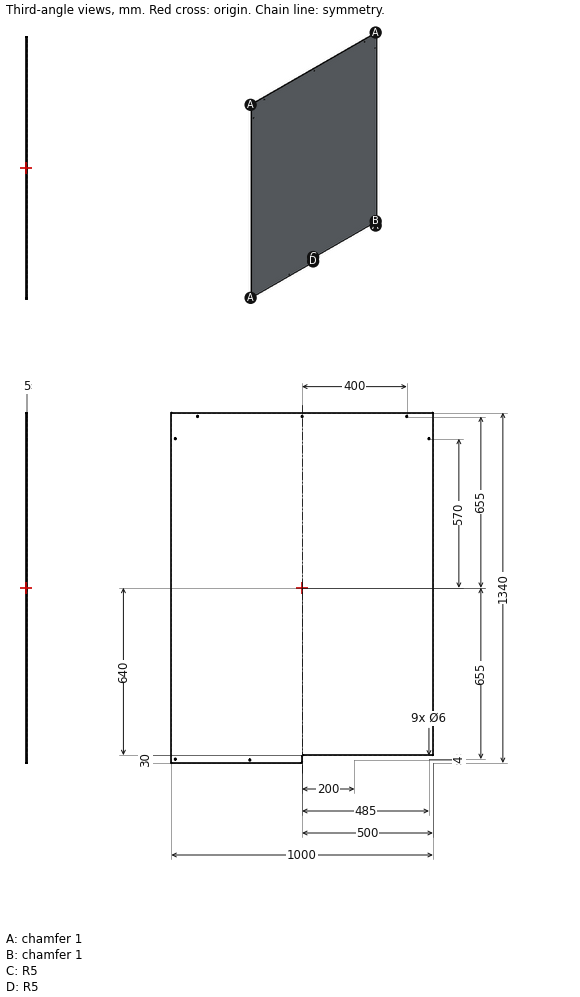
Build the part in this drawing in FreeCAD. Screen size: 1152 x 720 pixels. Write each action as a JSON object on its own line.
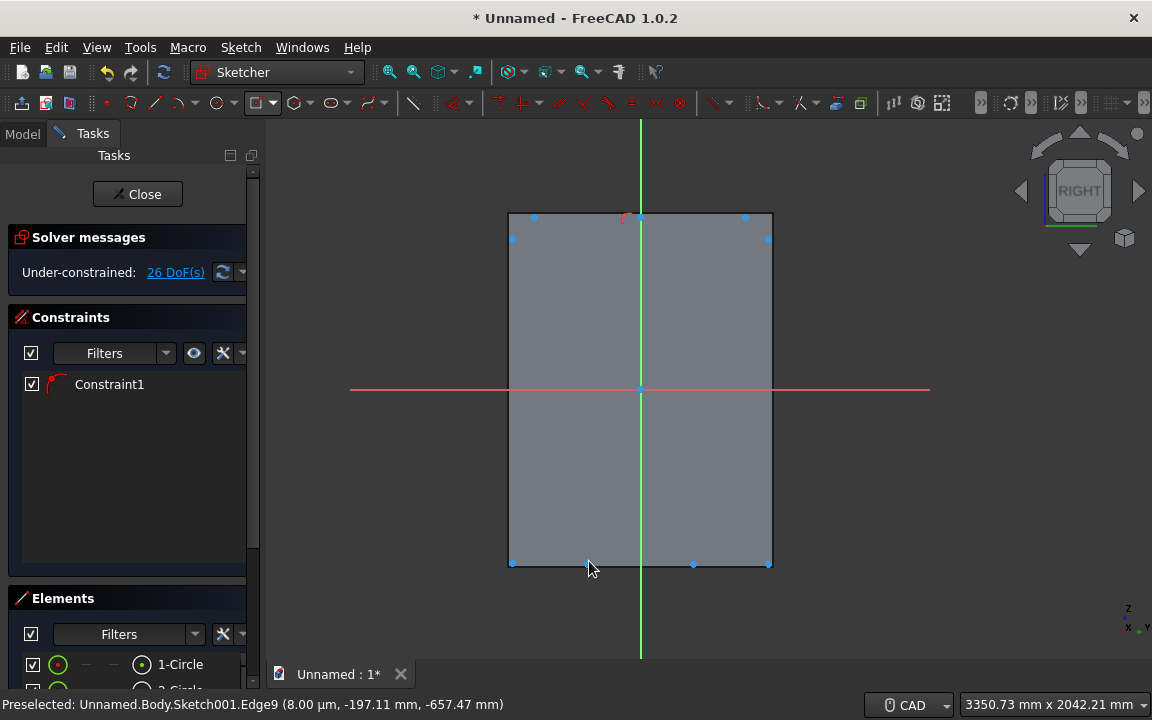
{"action": "scroll", "coordinate": [770, 563], "scroll_direction": "up", "scroll_amount": 10}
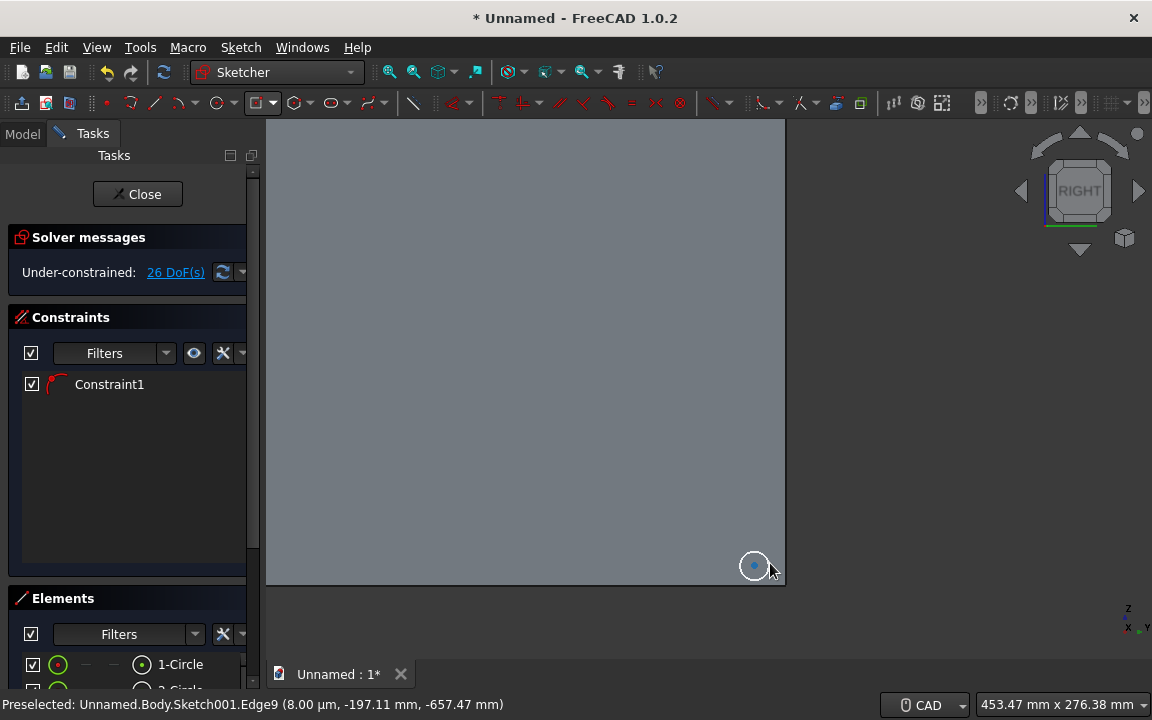
{"action": "left_click", "coordinate": [764, 556]}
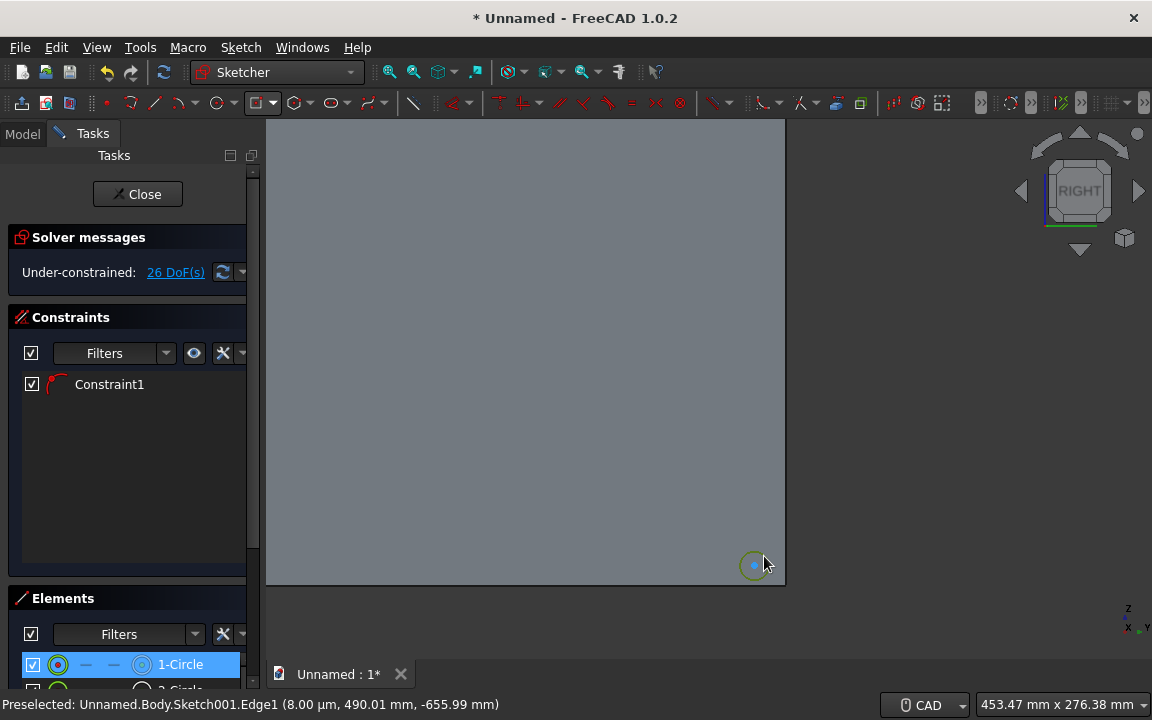
{"action": "scroll", "coordinate": [771, 562], "scroll_direction": "down", "scroll_amount": 10}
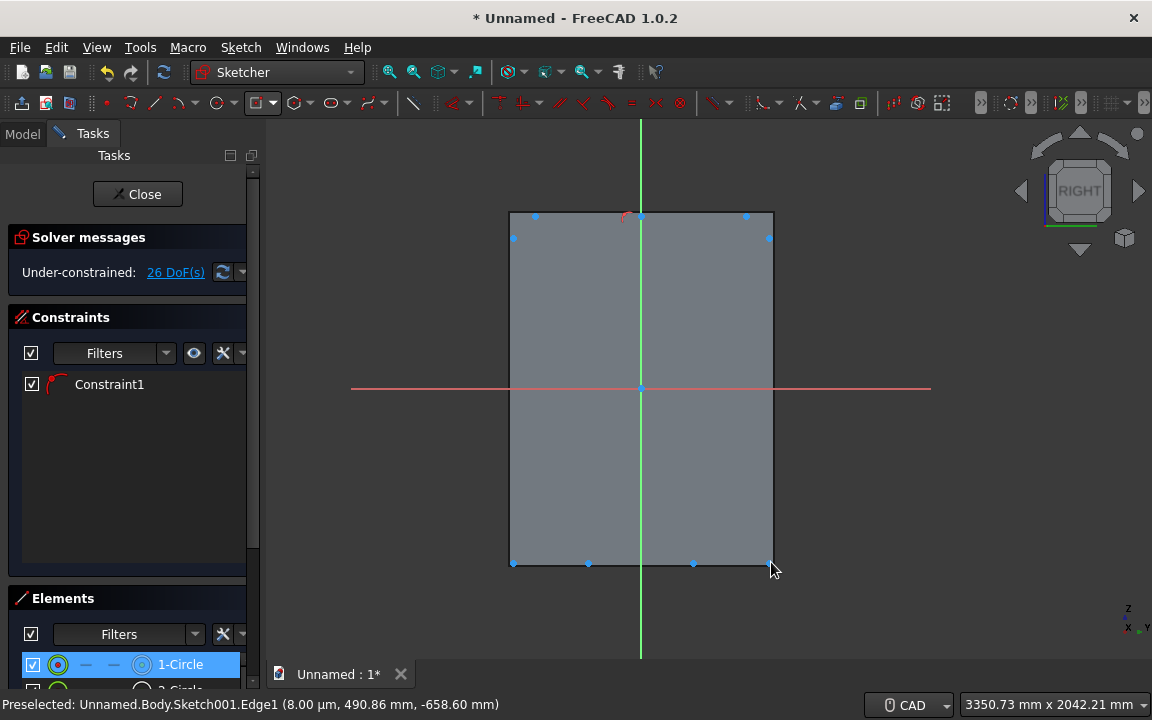
{"action": "scroll", "coordinate": [515, 562], "scroll_direction": "up", "scroll_amount": 11}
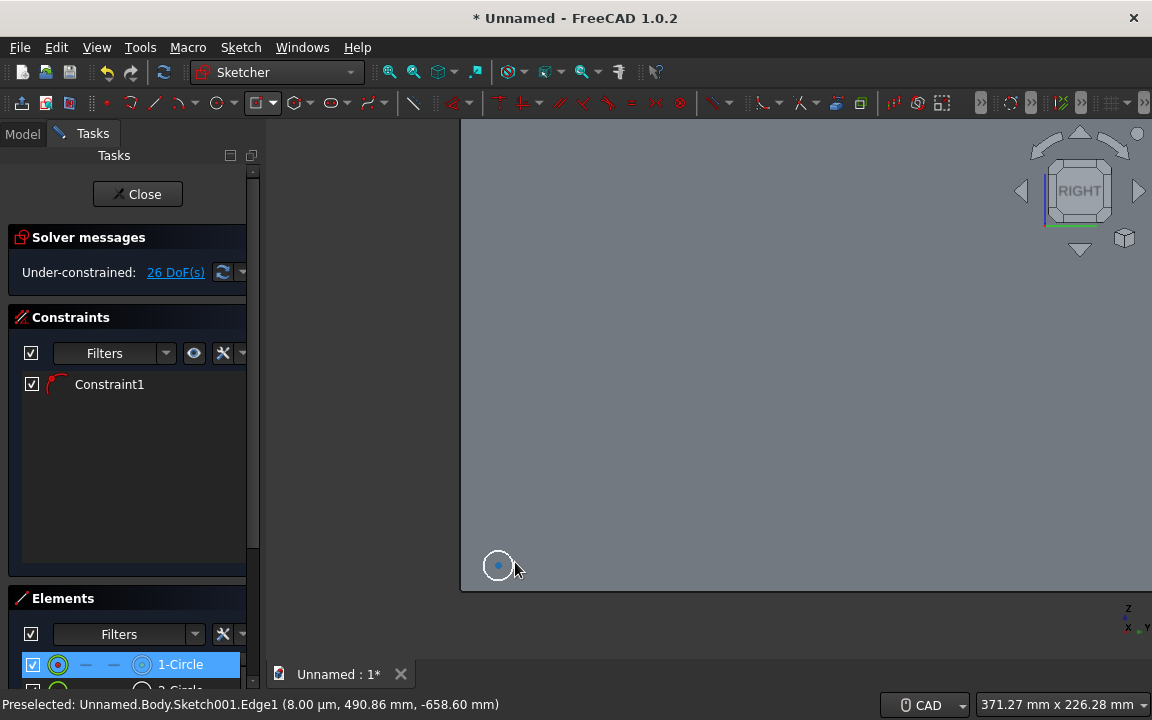
{"action": "left_click", "coordinate": [509, 555]}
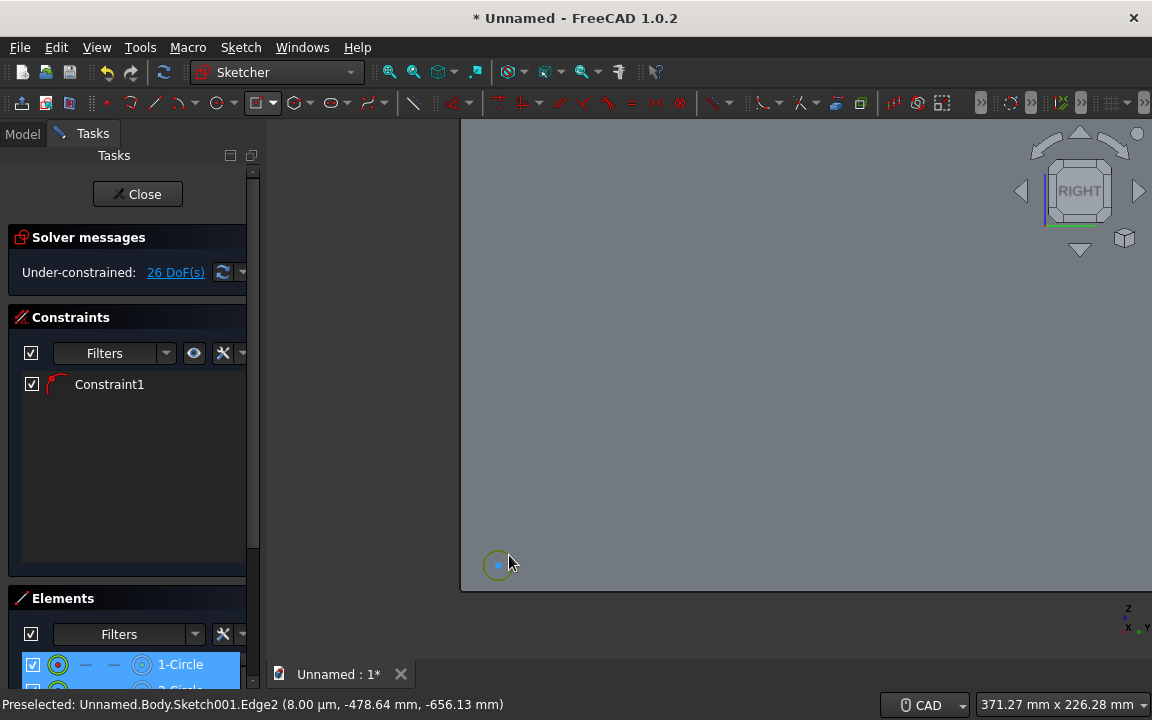
{"action": "scroll", "coordinate": [514, 562], "scroll_direction": "down", "scroll_amount": 11}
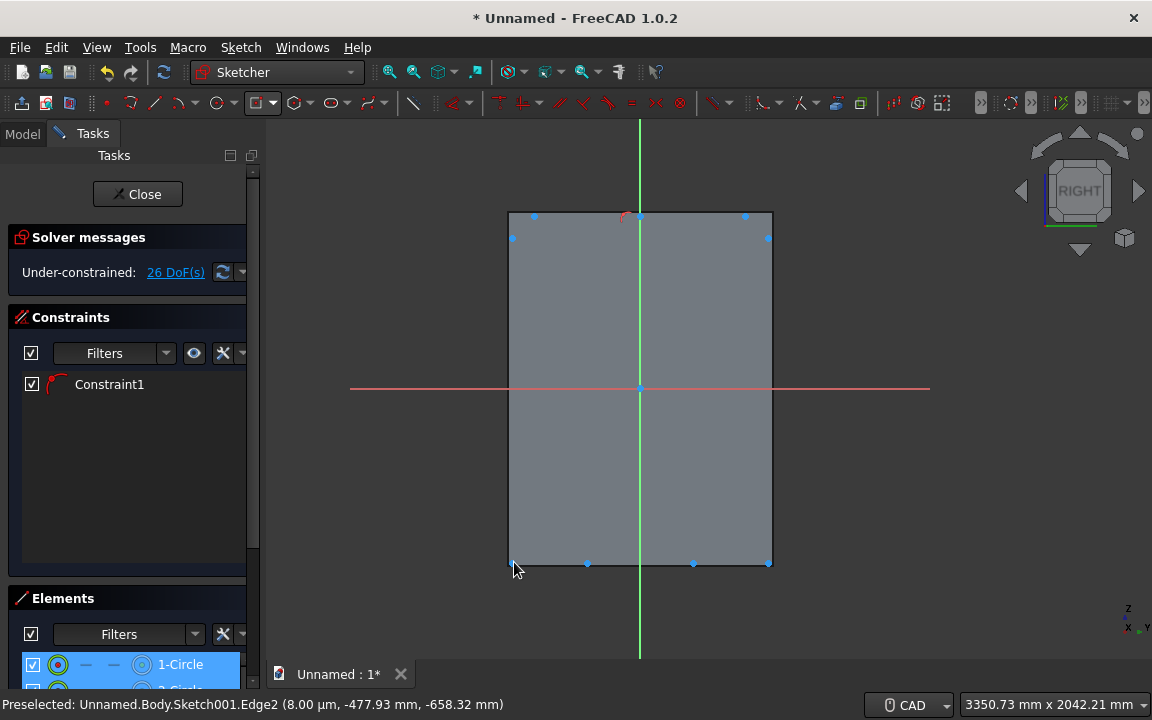
{"action": "scroll", "coordinate": [769, 238], "scroll_direction": "up", "scroll_amount": 11}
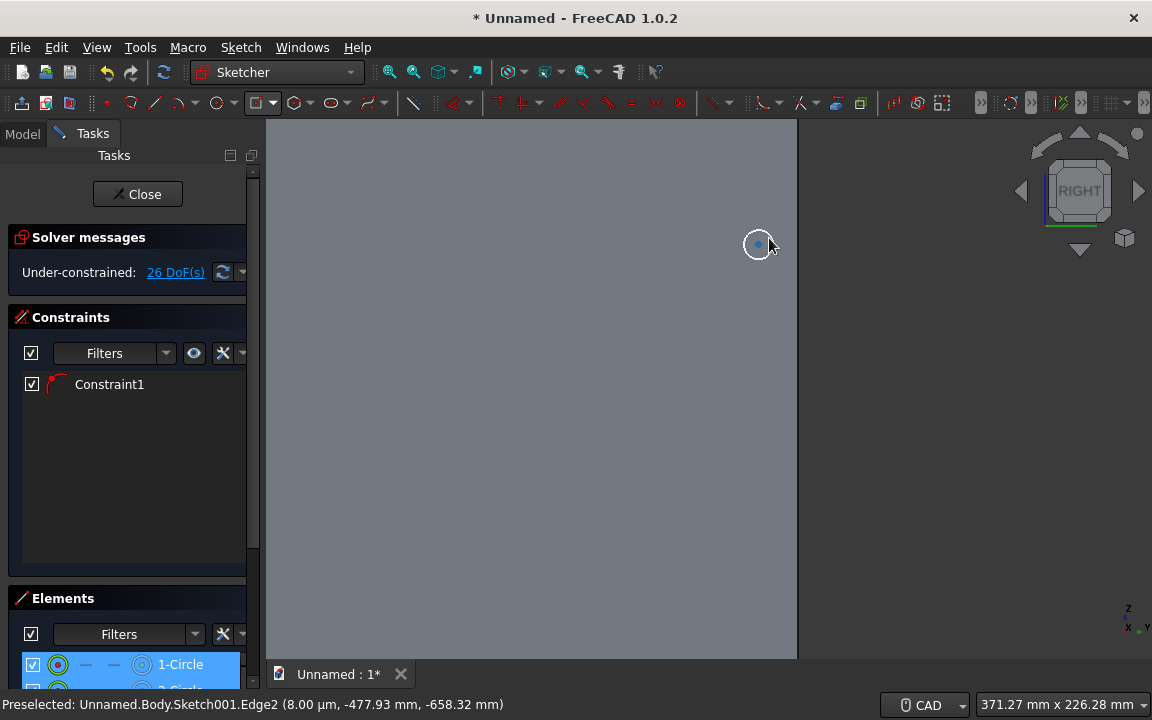
{"action": "left_click", "coordinate": [769, 234]}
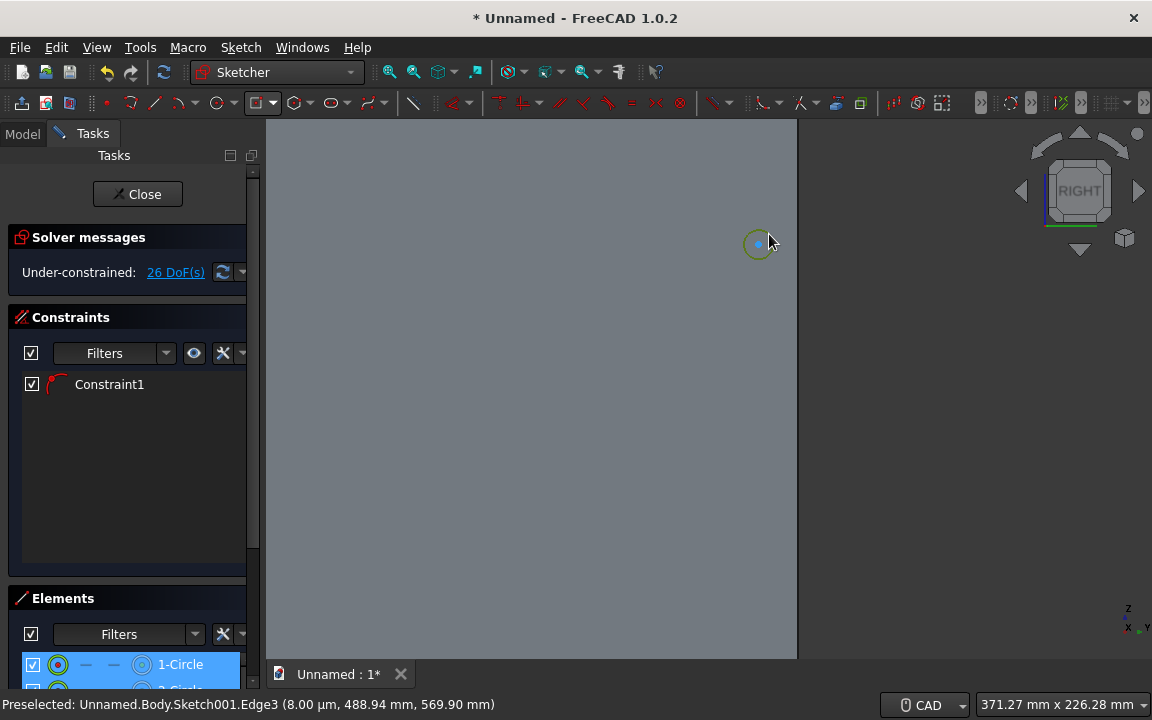
{"action": "scroll", "coordinate": [770, 238], "scroll_direction": "down", "scroll_amount": 11}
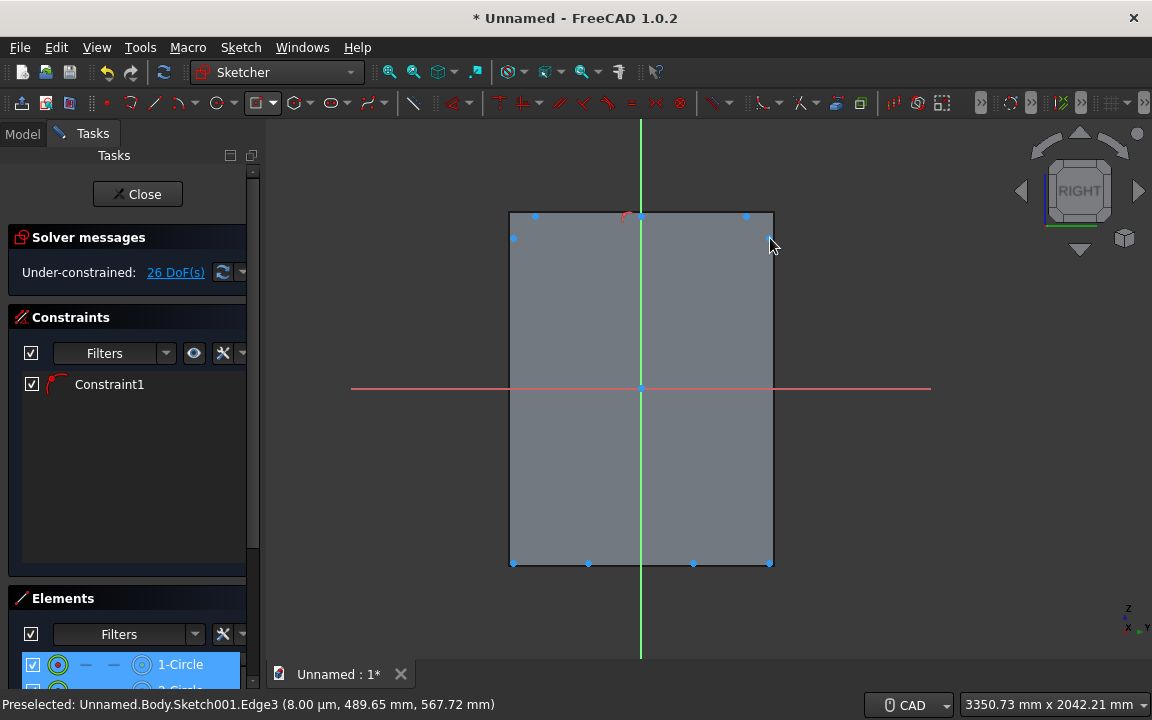
{"action": "scroll", "coordinate": [748, 215], "scroll_direction": "up", "scroll_amount": 11}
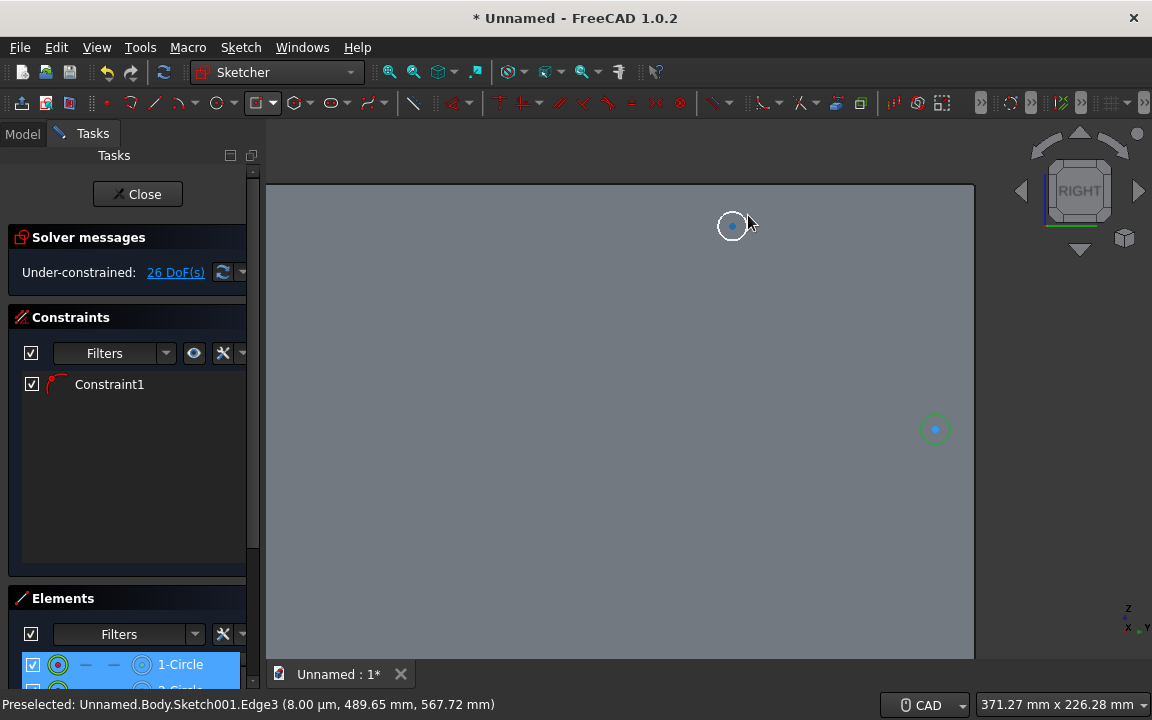
{"action": "left_click", "coordinate": [743, 216]}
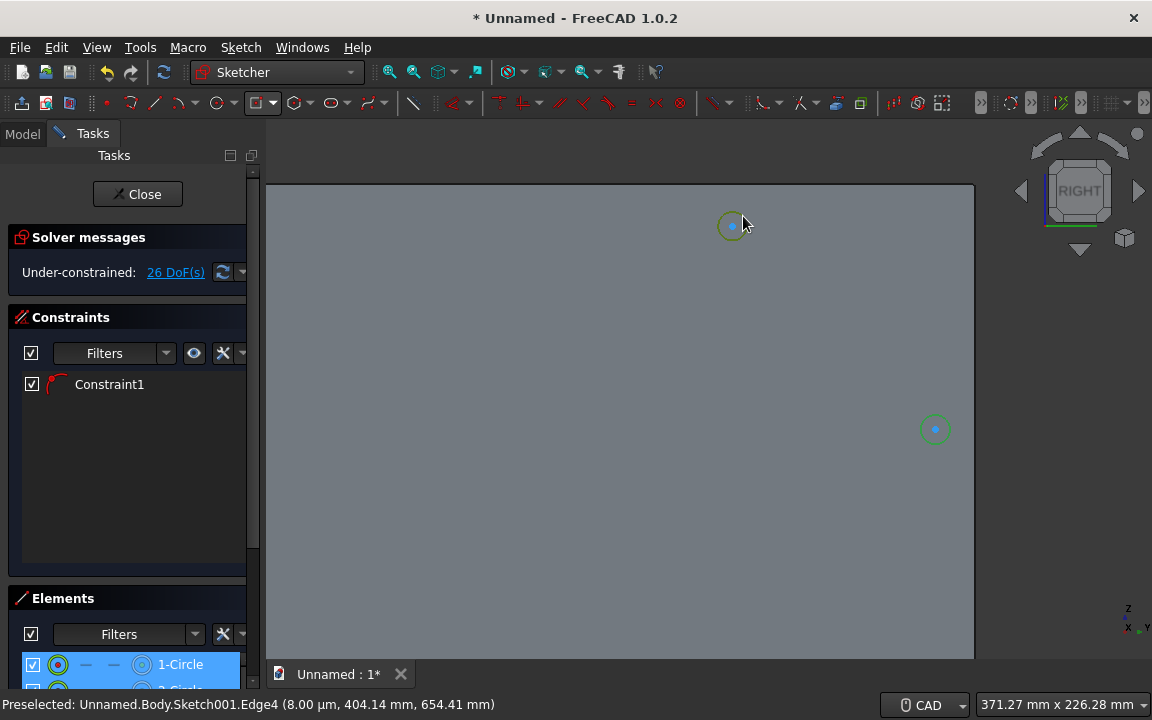
{"action": "scroll", "coordinate": [748, 215], "scroll_direction": "down", "scroll_amount": 11}